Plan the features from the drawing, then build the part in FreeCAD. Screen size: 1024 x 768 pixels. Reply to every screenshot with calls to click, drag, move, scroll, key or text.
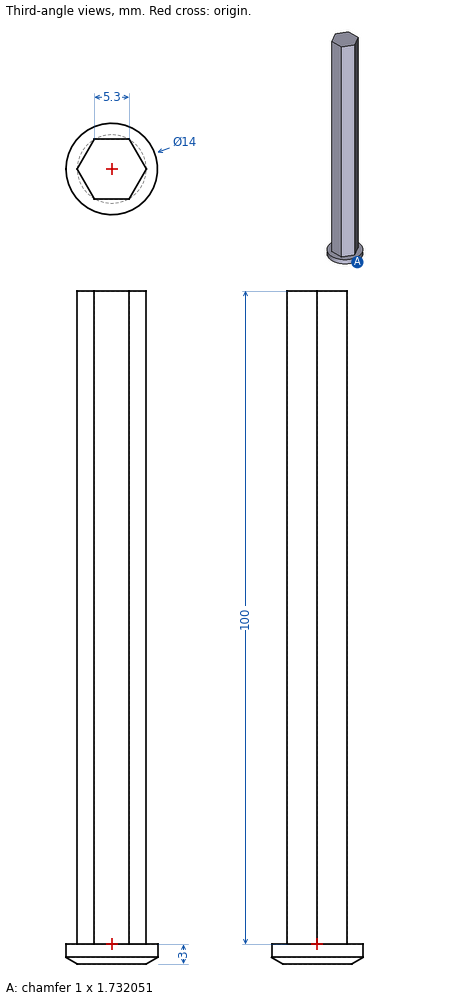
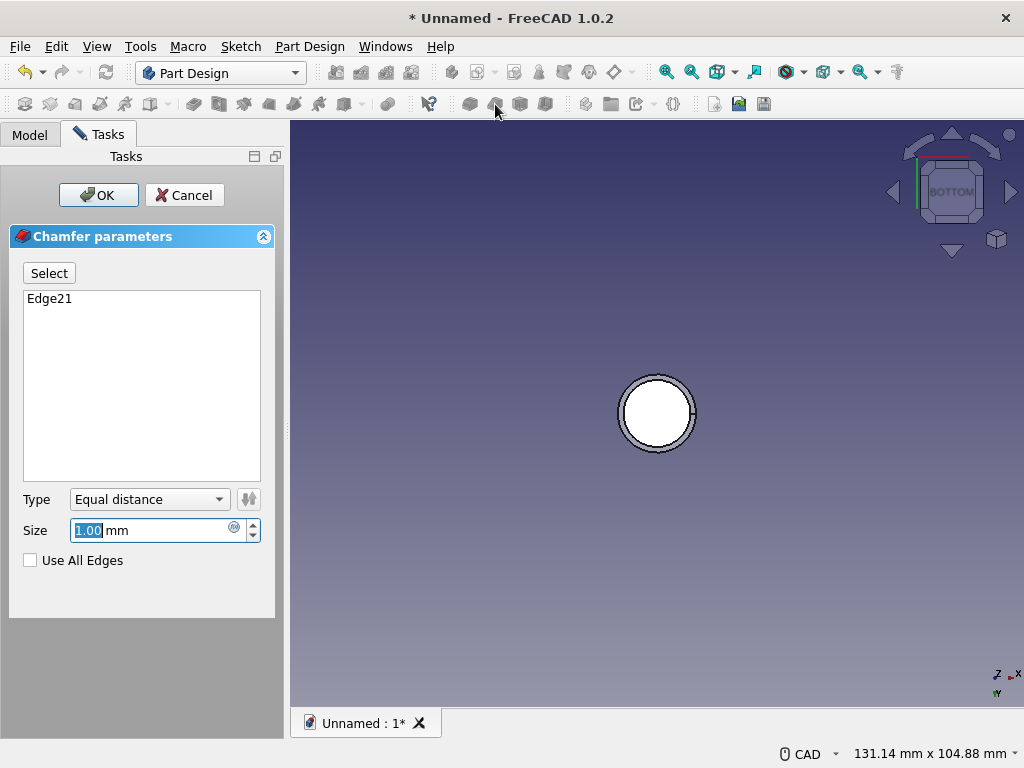
text(1)
key(Tab)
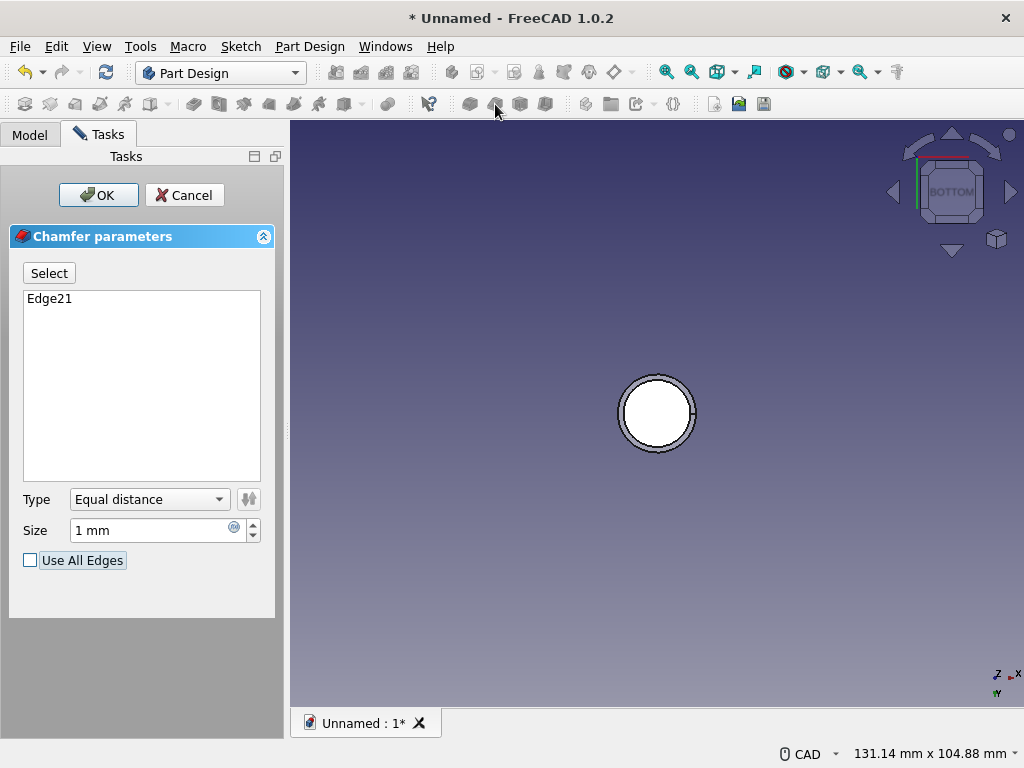
click(150, 500)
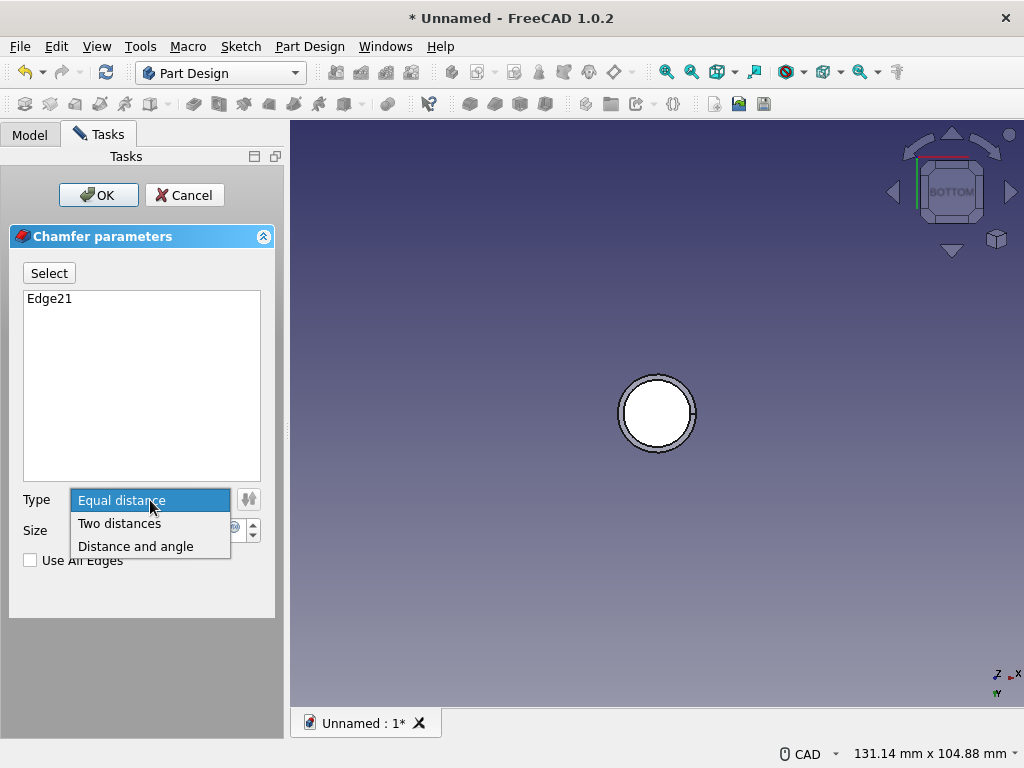
click(148, 524)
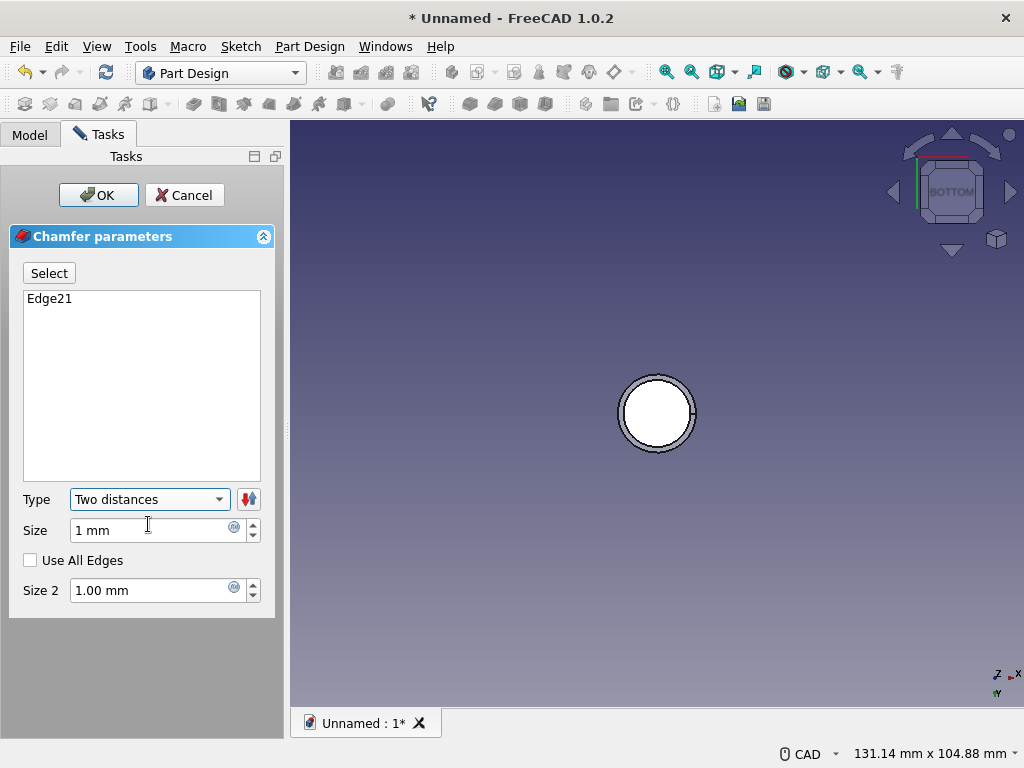
triple_click(158, 590)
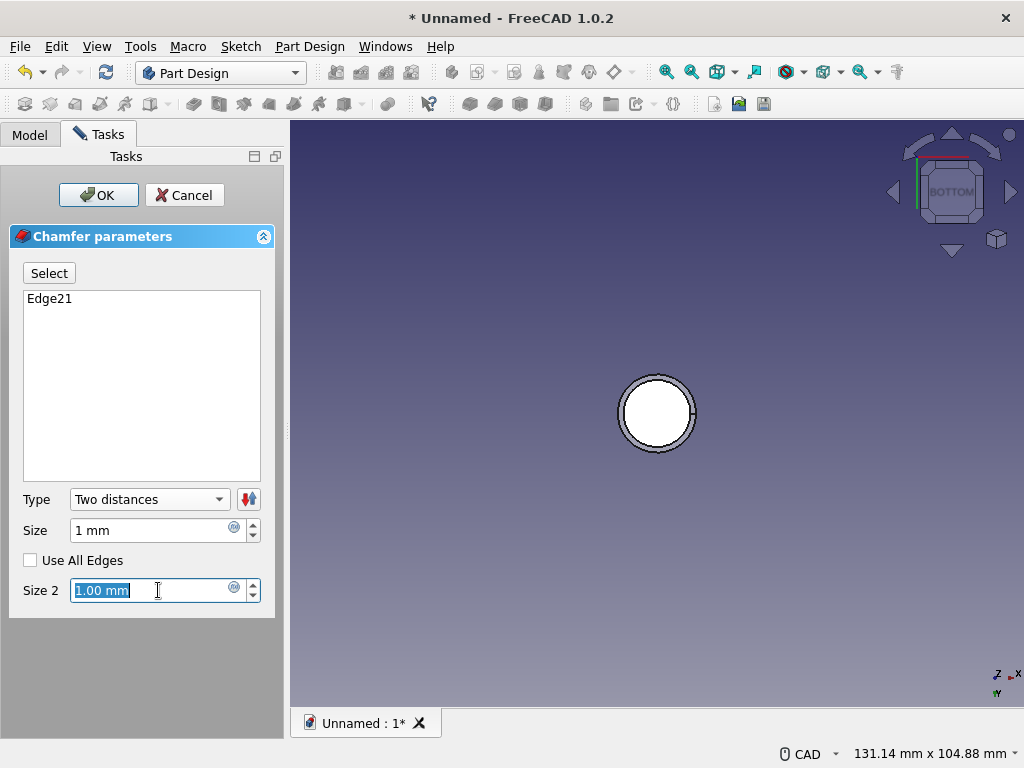
text(1.732051)
key(Tab)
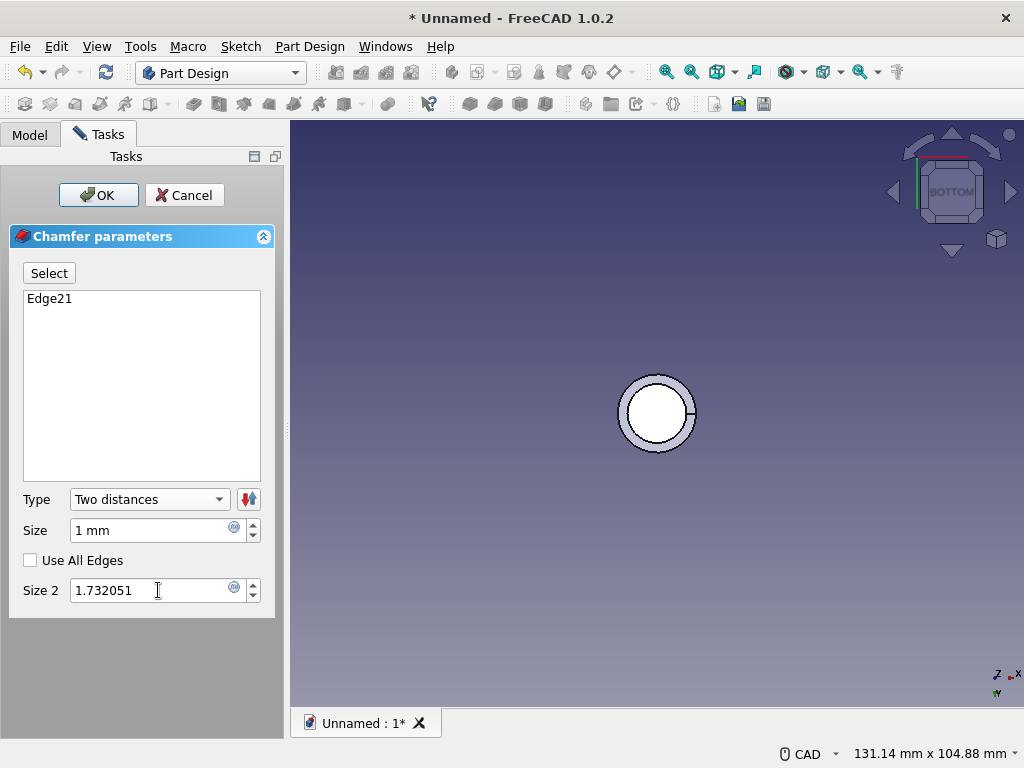
click(99, 195)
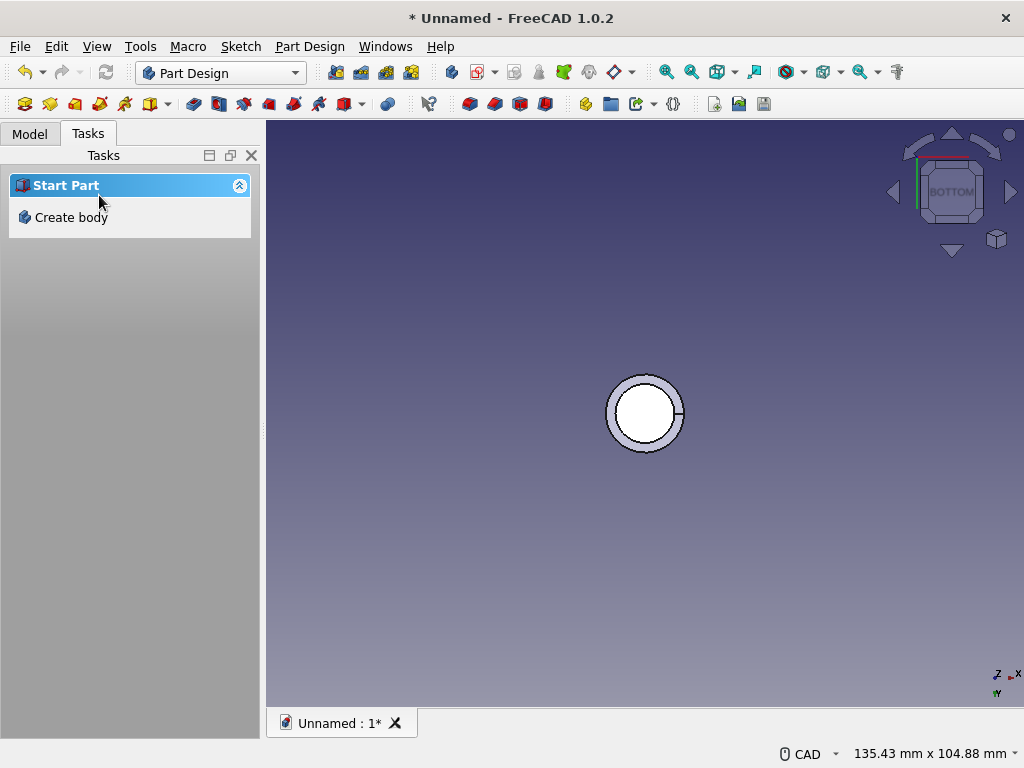
key(0)